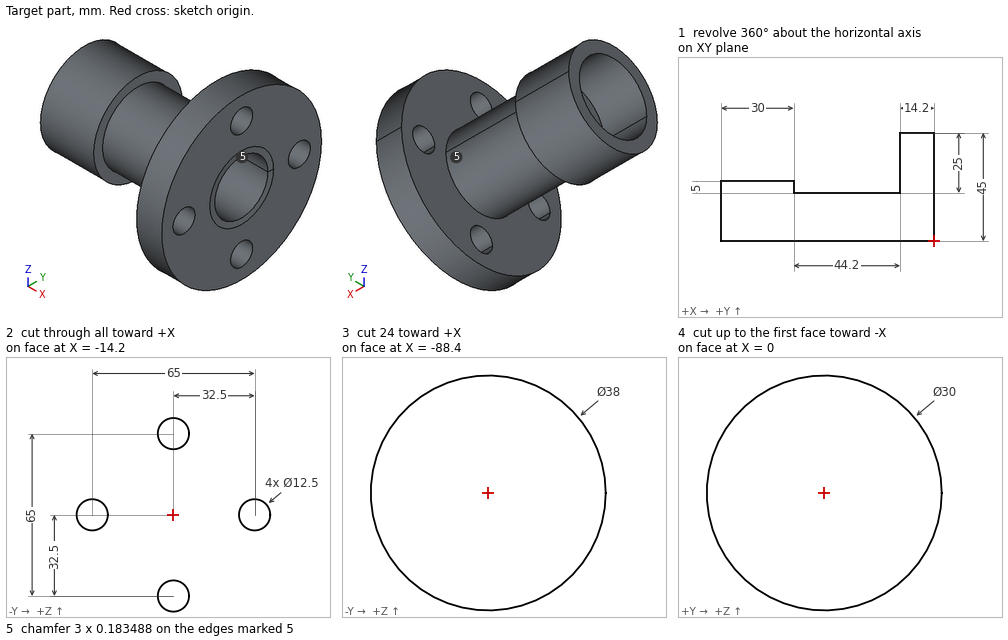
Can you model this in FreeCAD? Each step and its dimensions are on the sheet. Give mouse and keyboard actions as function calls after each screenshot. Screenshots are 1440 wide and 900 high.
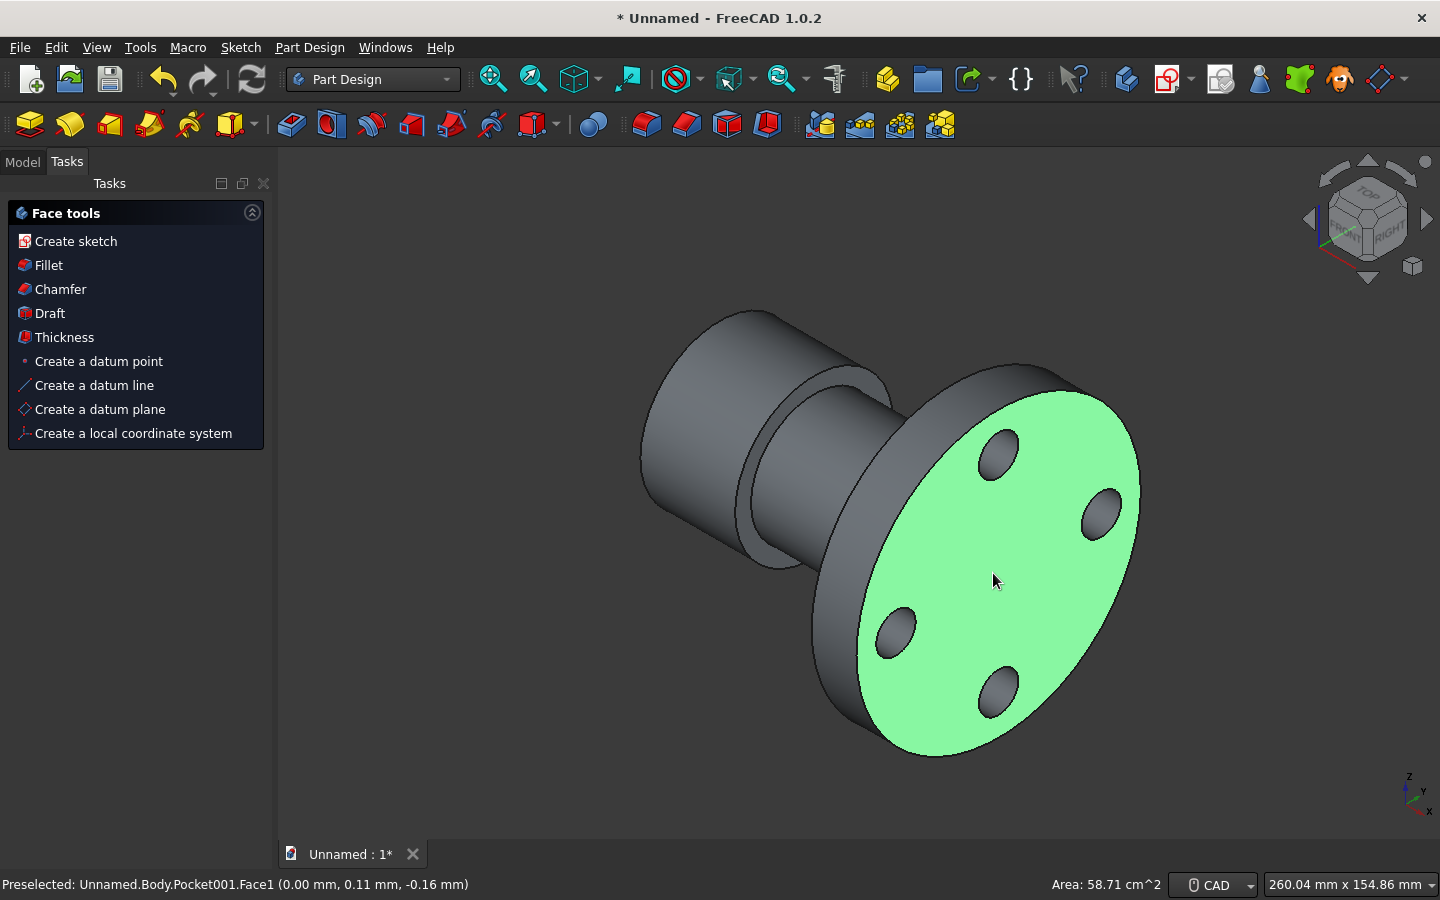
click(1168, 80)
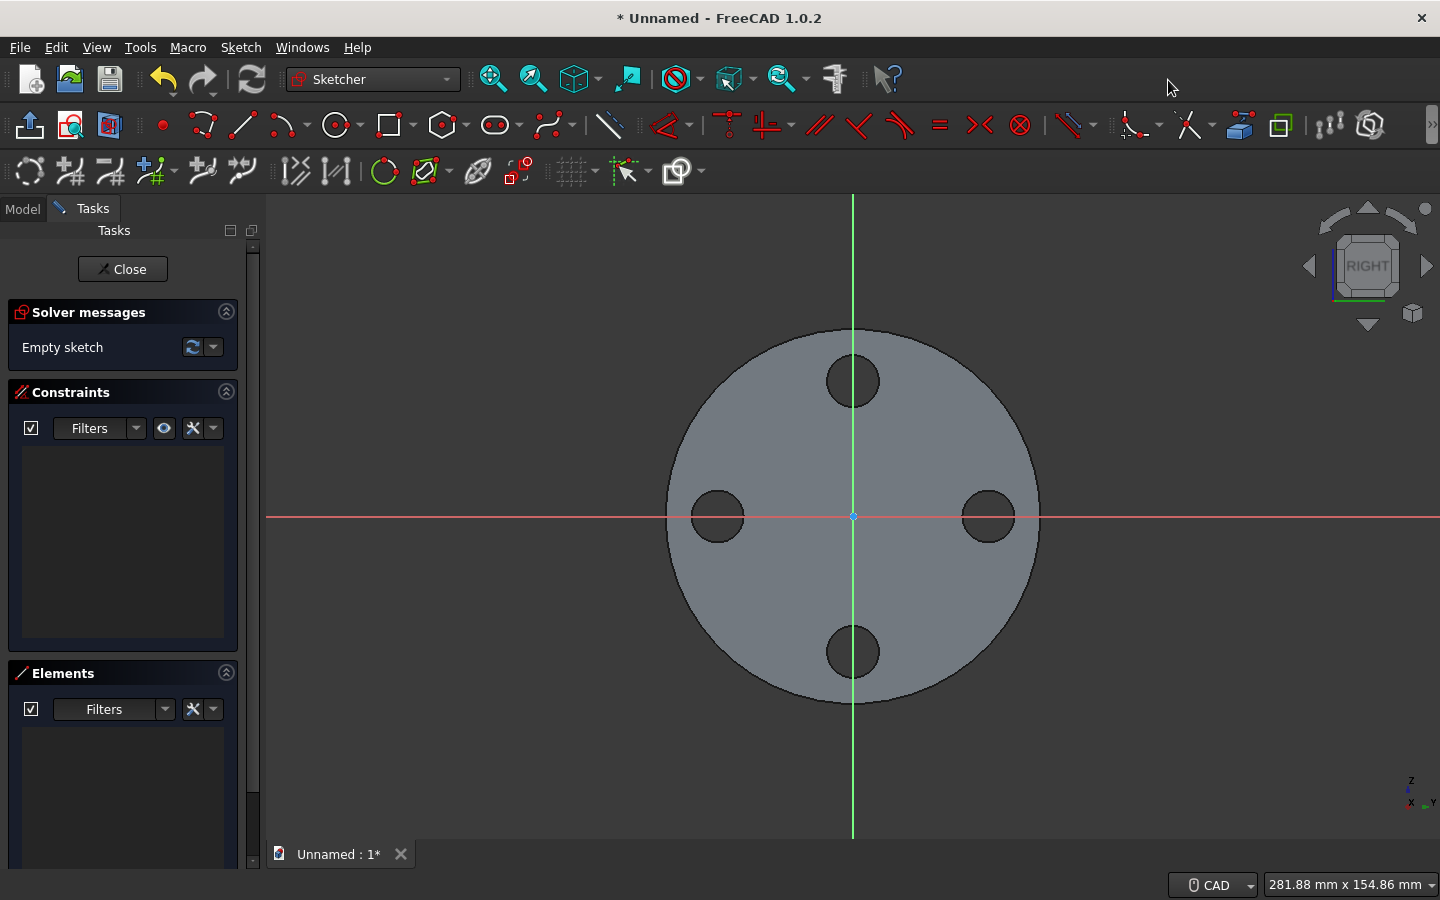
scroll(883, 517, up, 6)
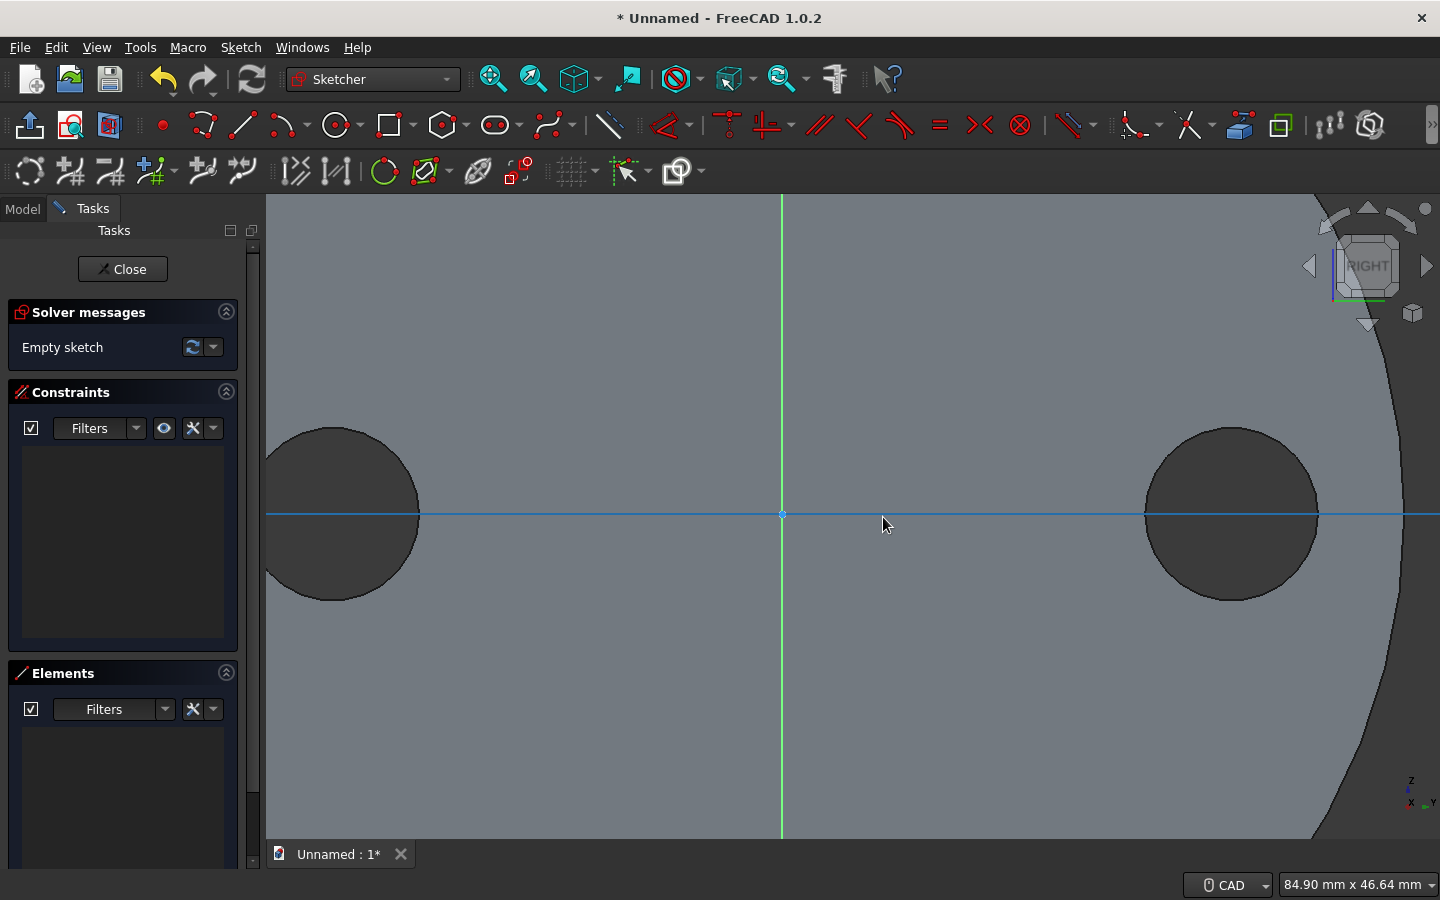
key(g)
key(c)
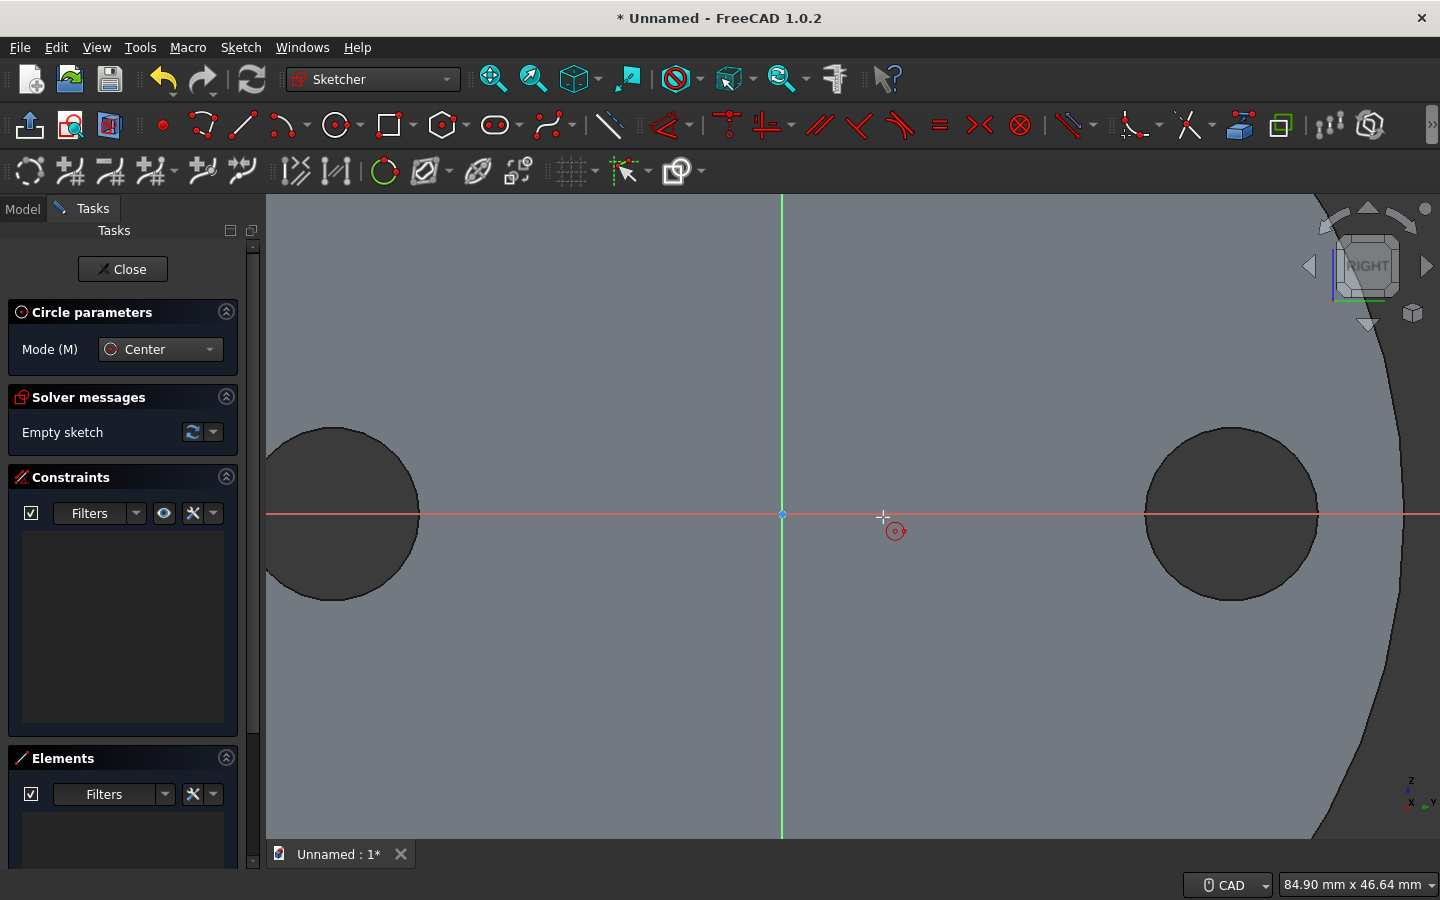
click(782, 514)
click(929, 368)
key(Escape)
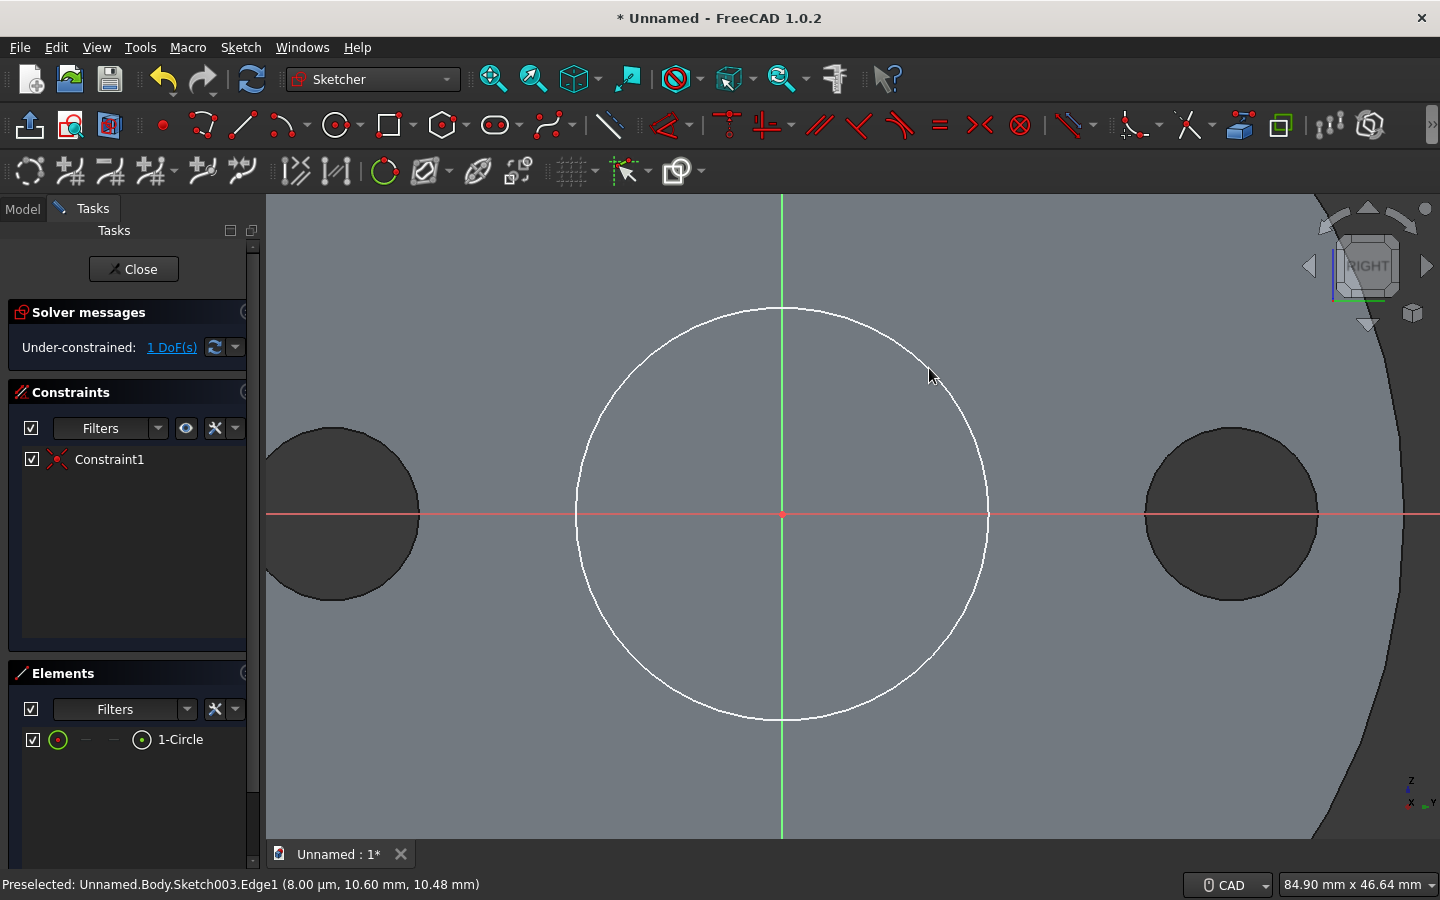
key(d)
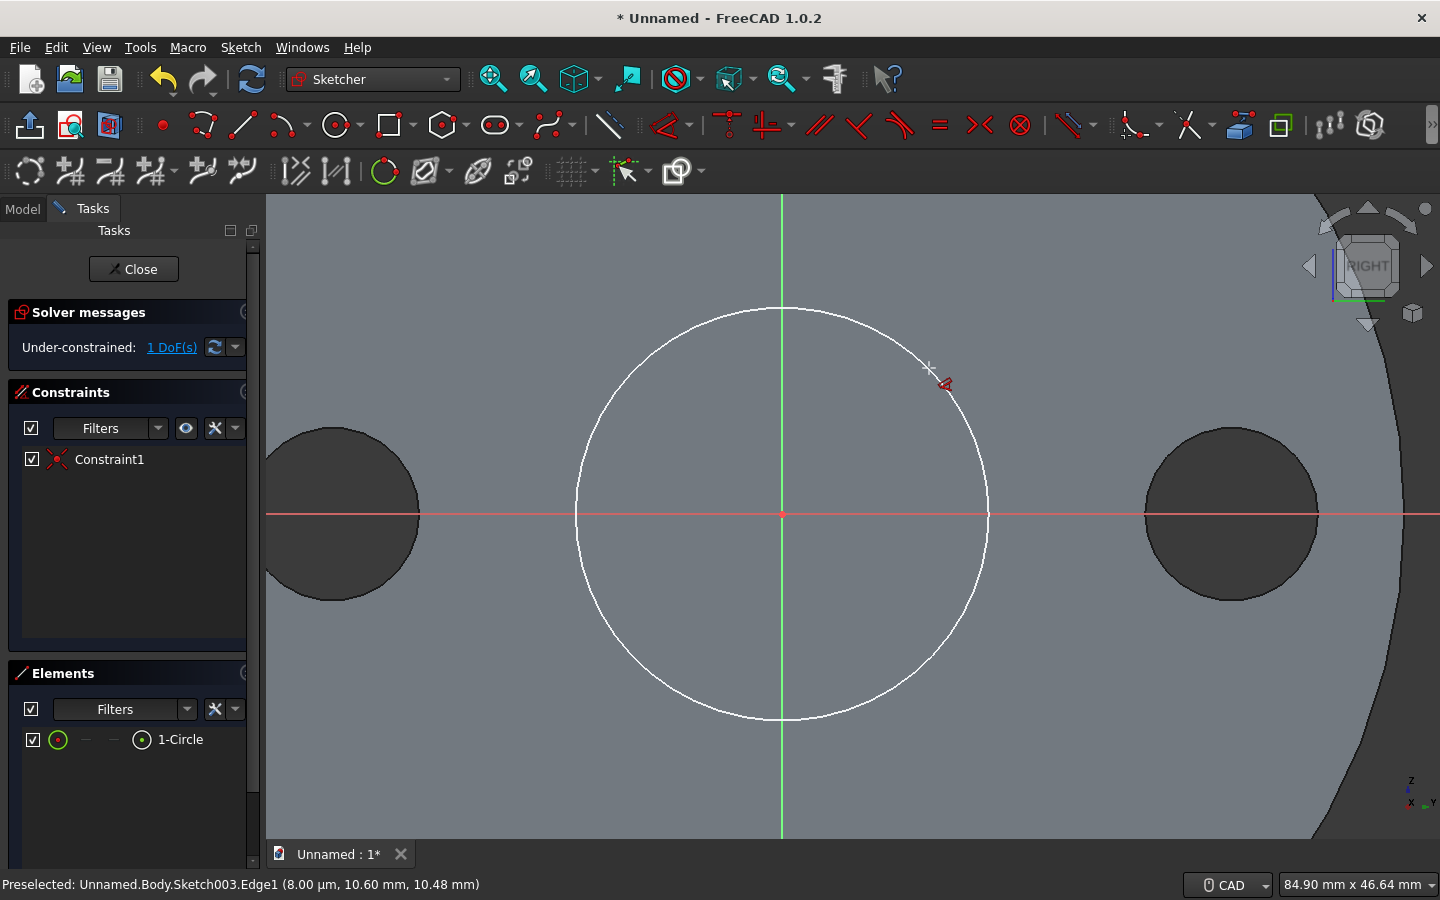
click(928, 368)
click(951, 345)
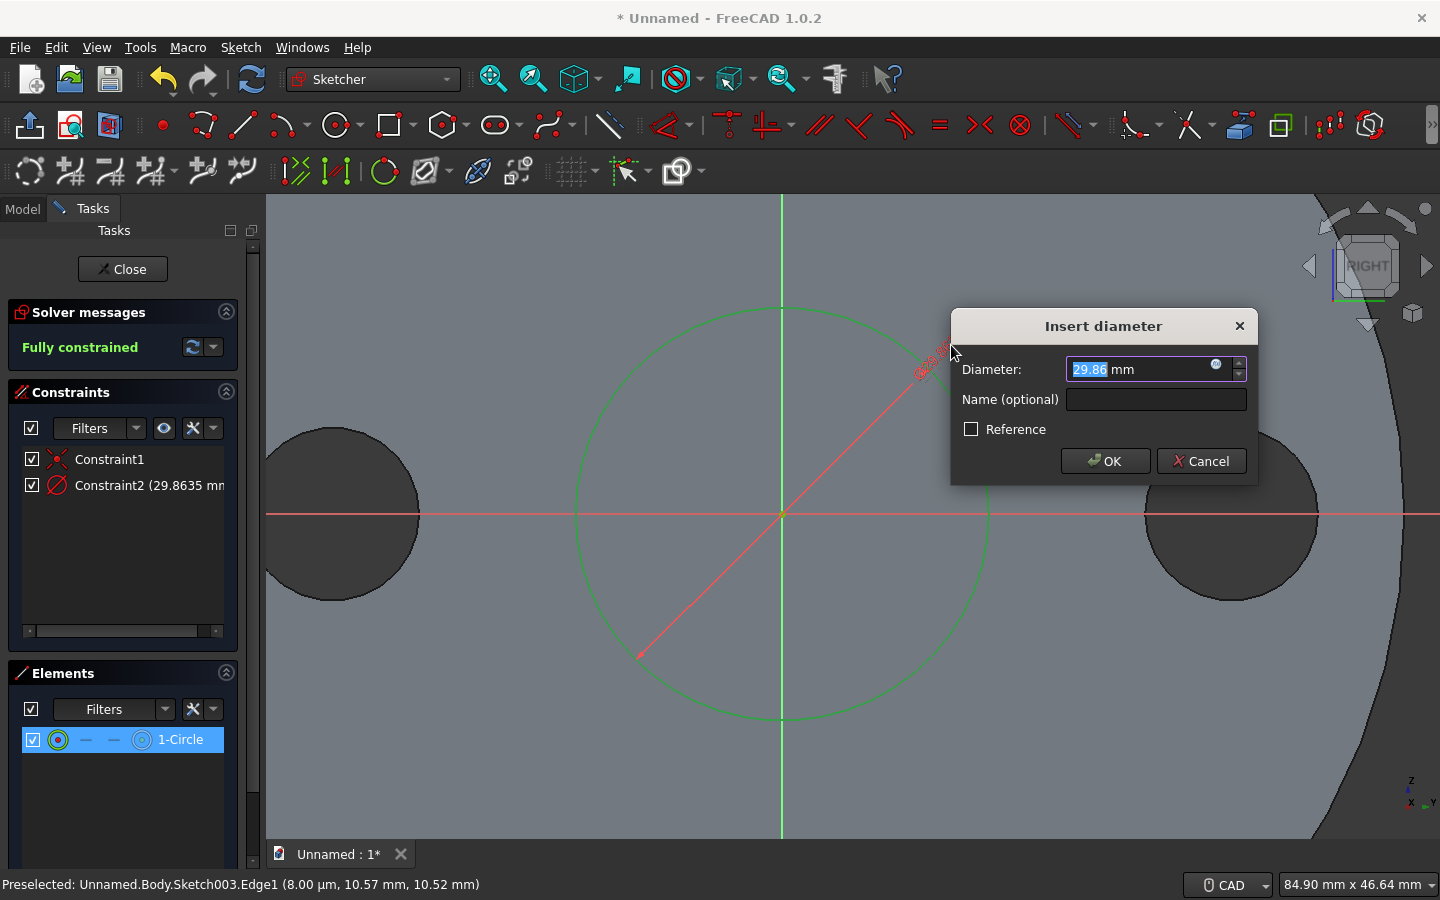
text(30)
key(Return)
key(Escape)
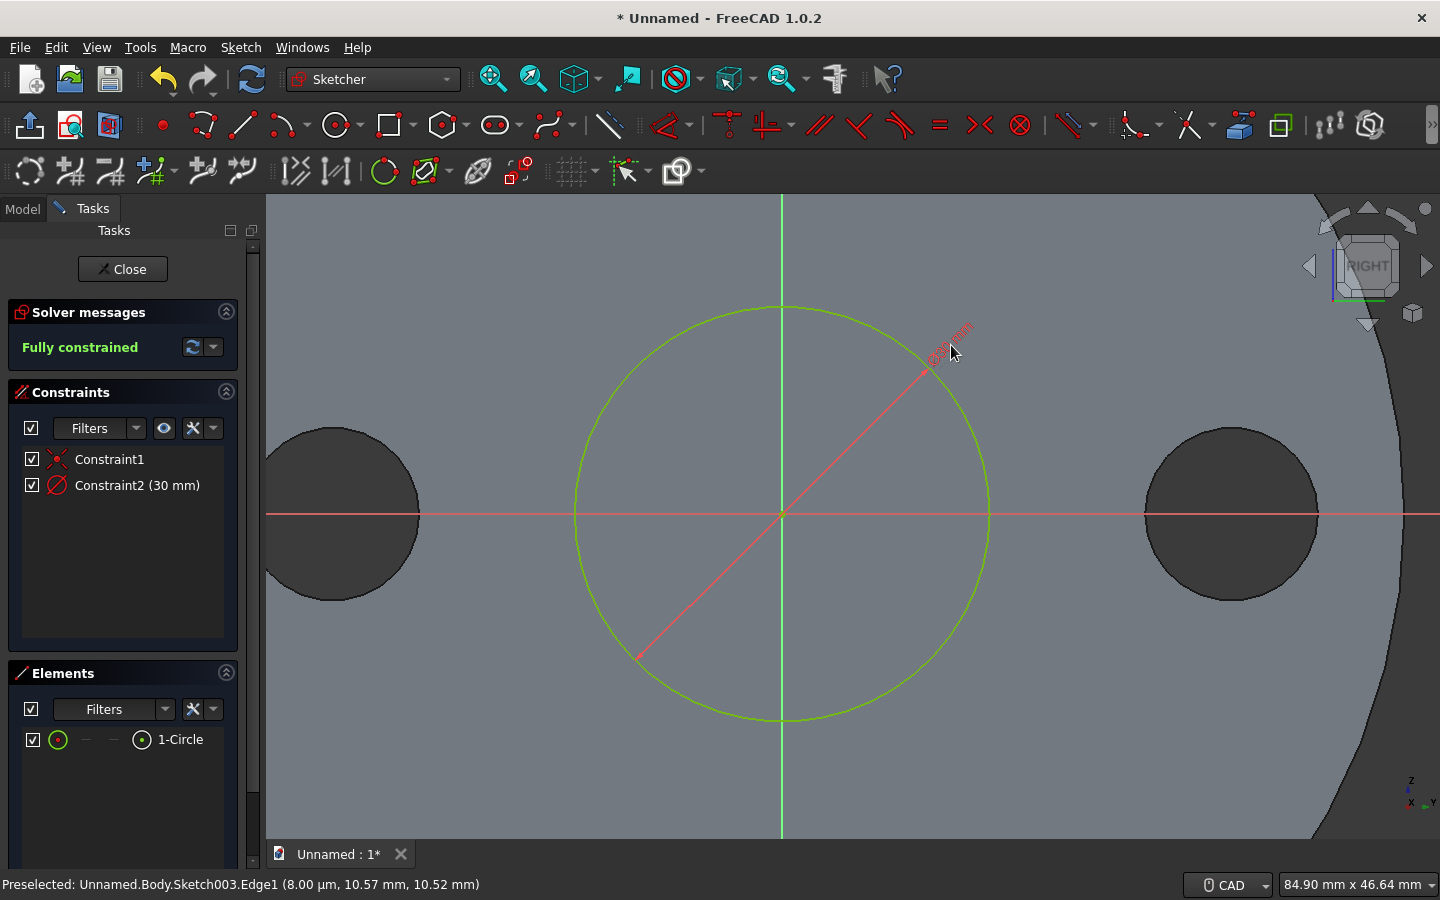
click(123, 269)